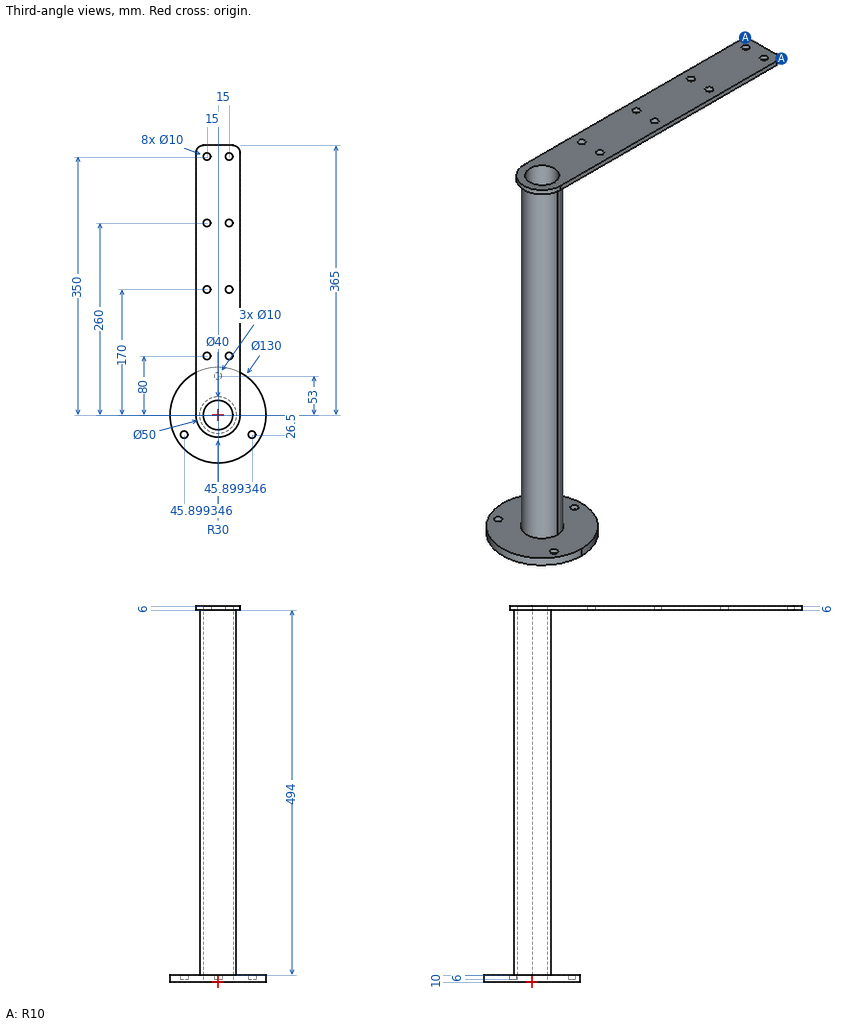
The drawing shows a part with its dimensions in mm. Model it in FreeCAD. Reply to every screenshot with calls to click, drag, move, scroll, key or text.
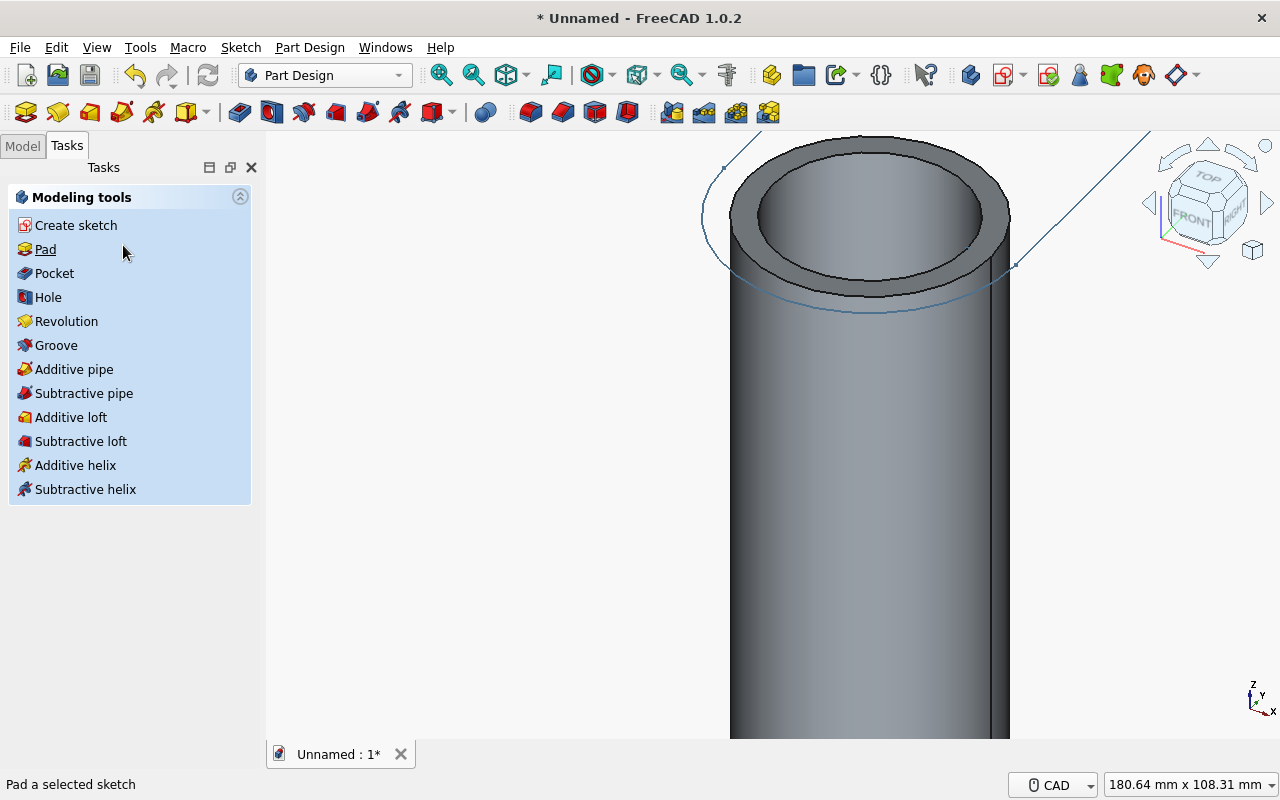
click(26, 112)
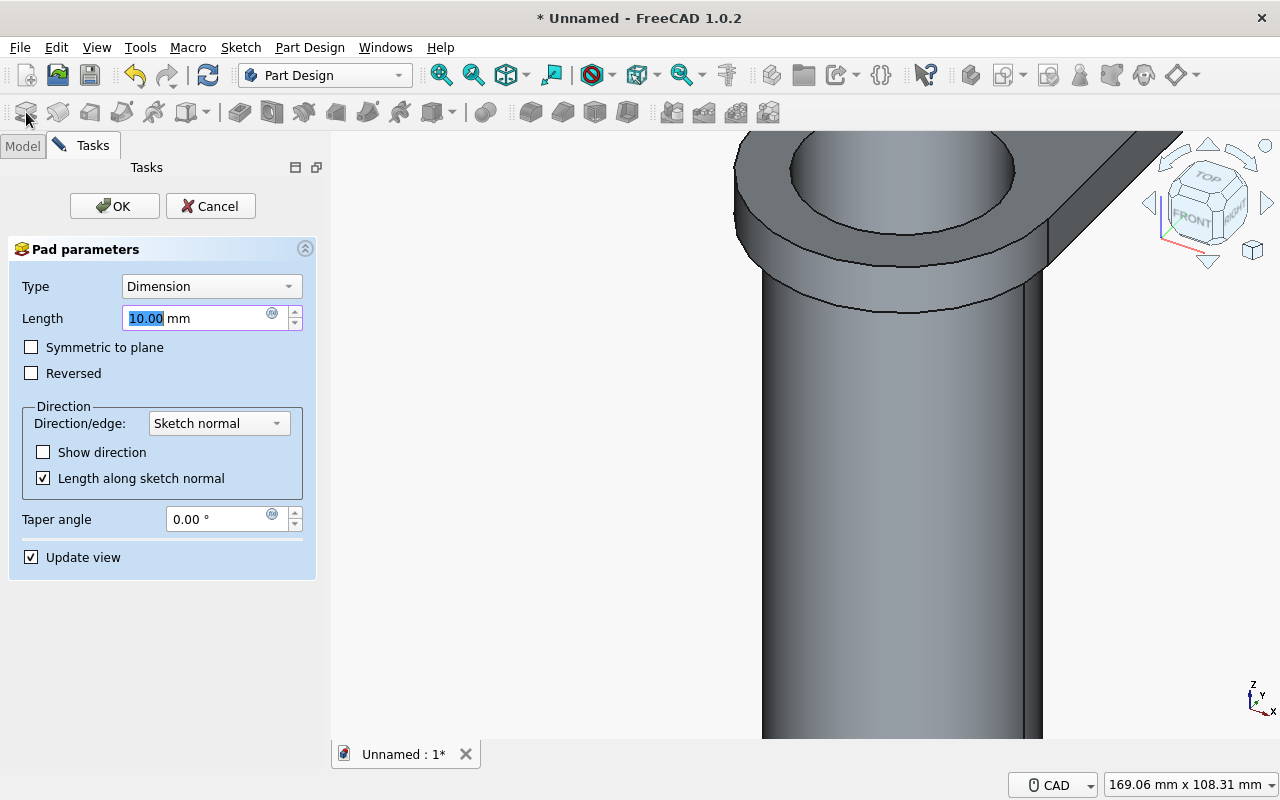
text(6)
key(Tab)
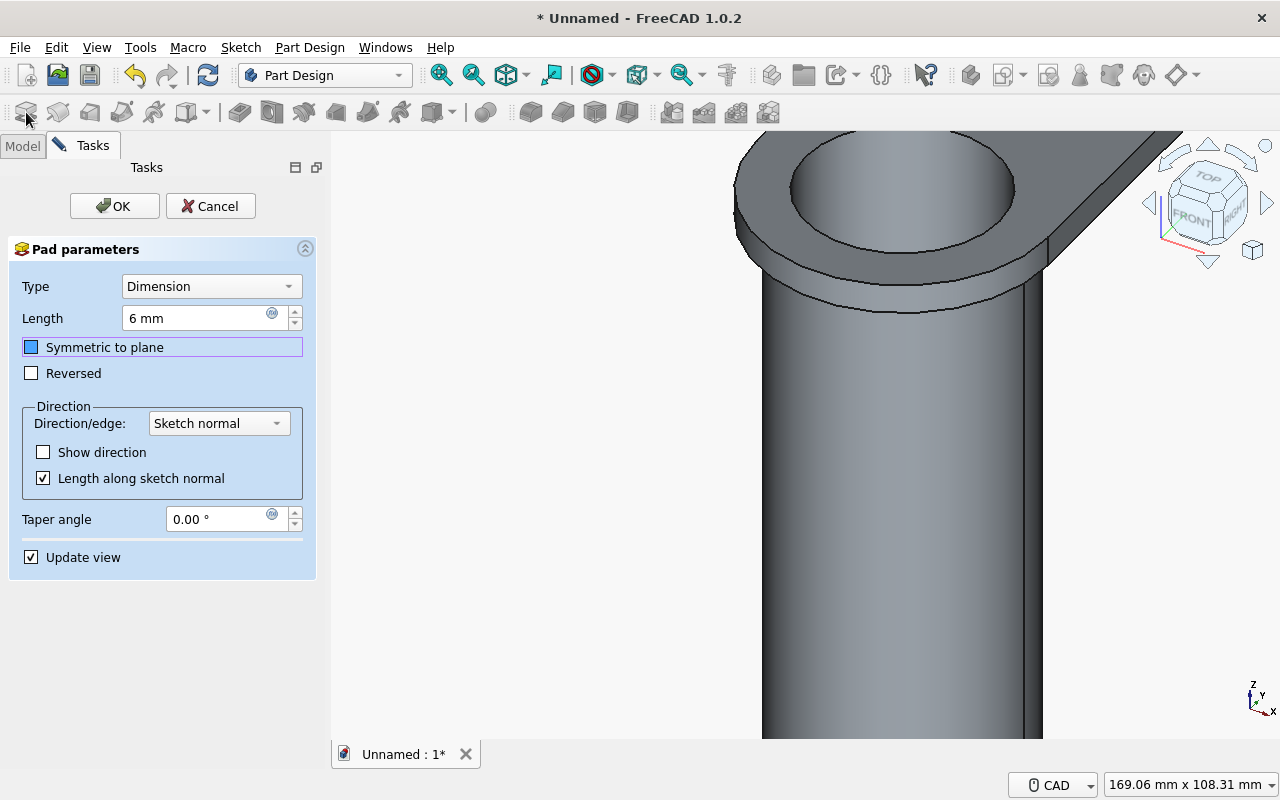
click(115, 206)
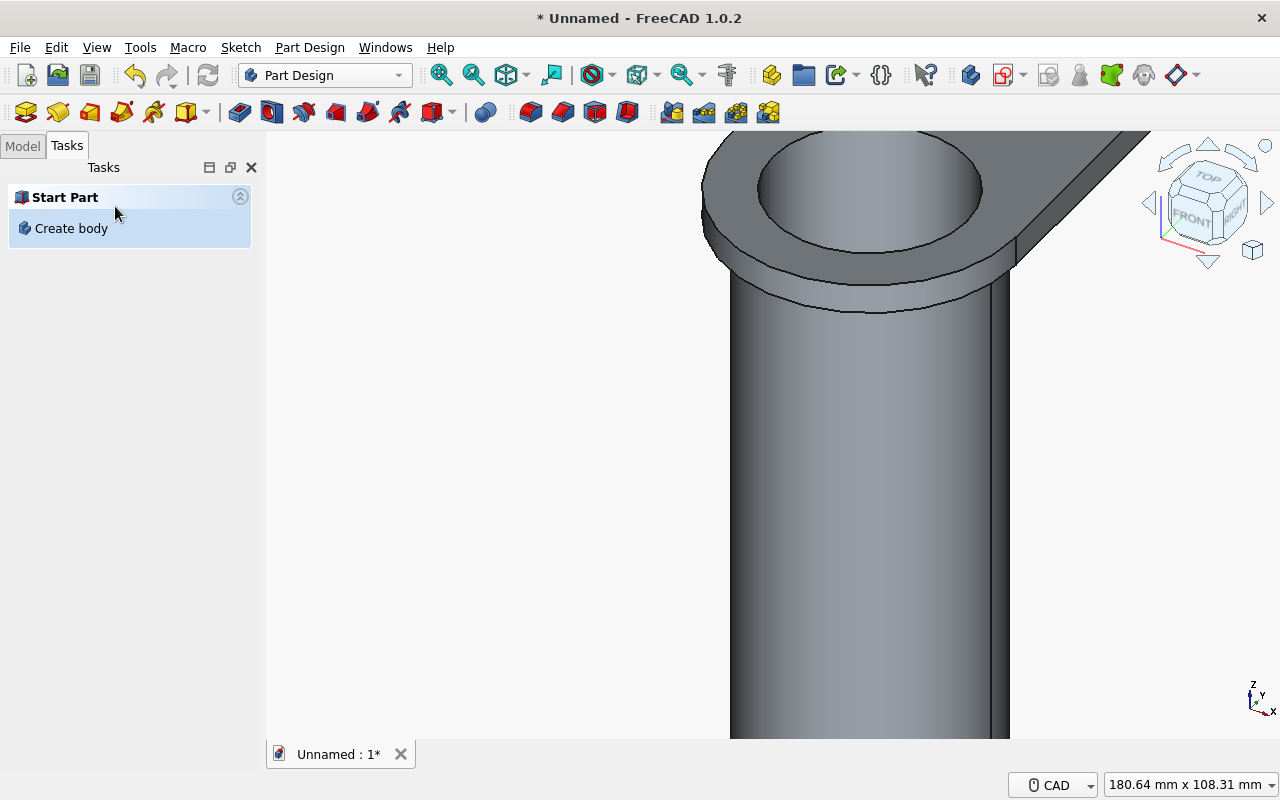
click(442, 76)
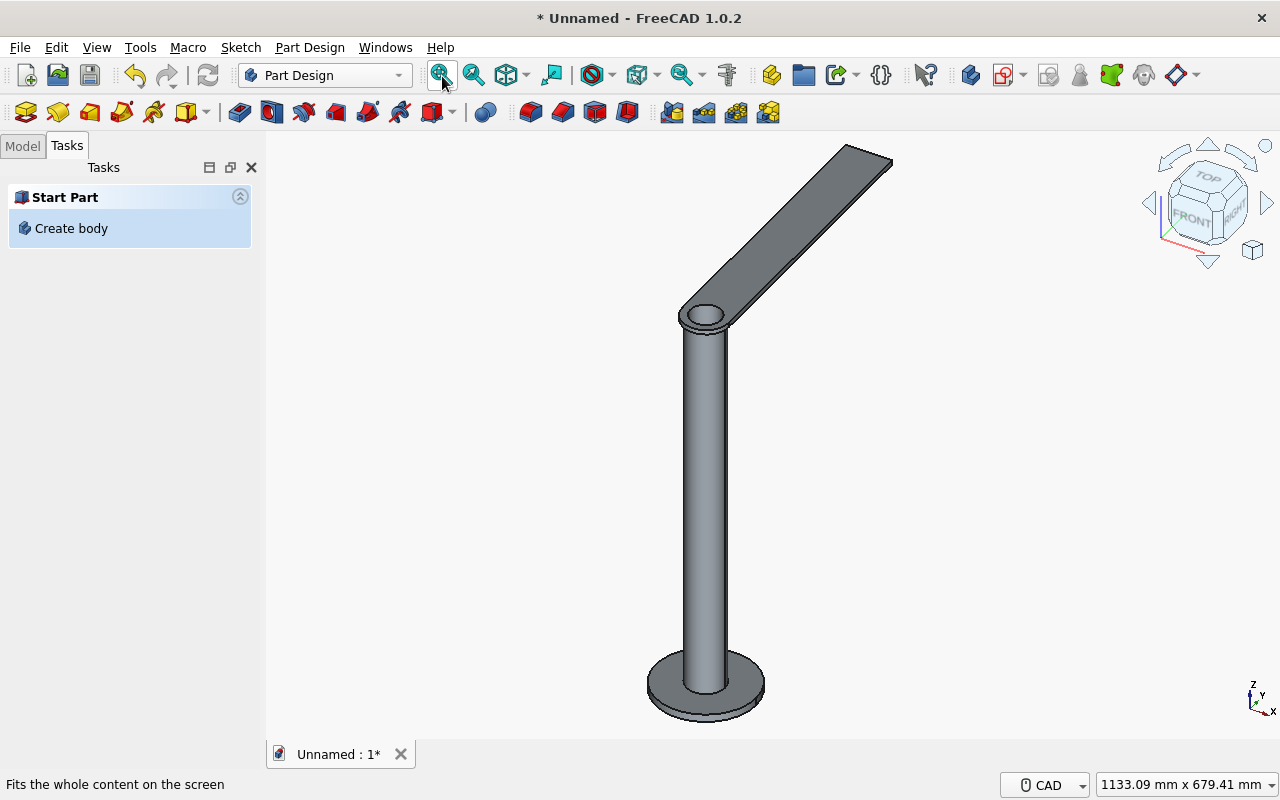
scroll(892, 161, up, 11)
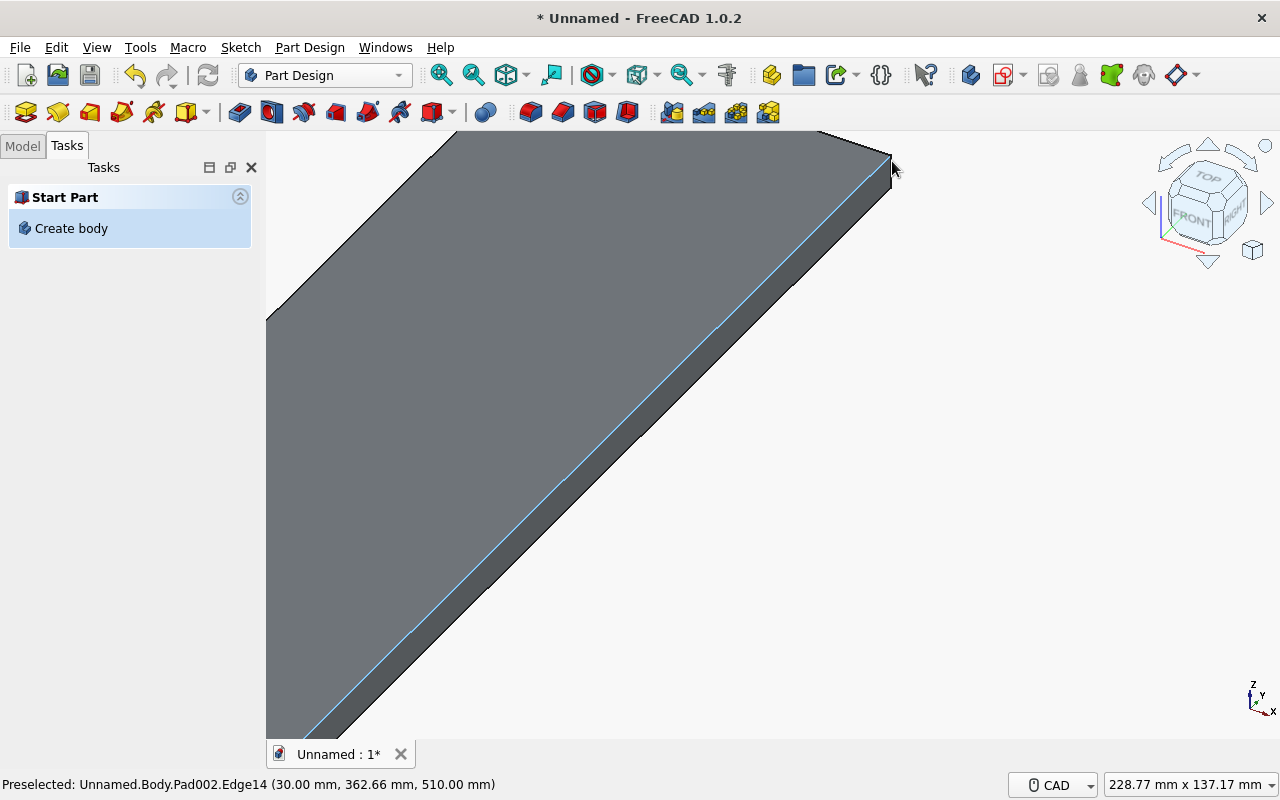
click(442, 76)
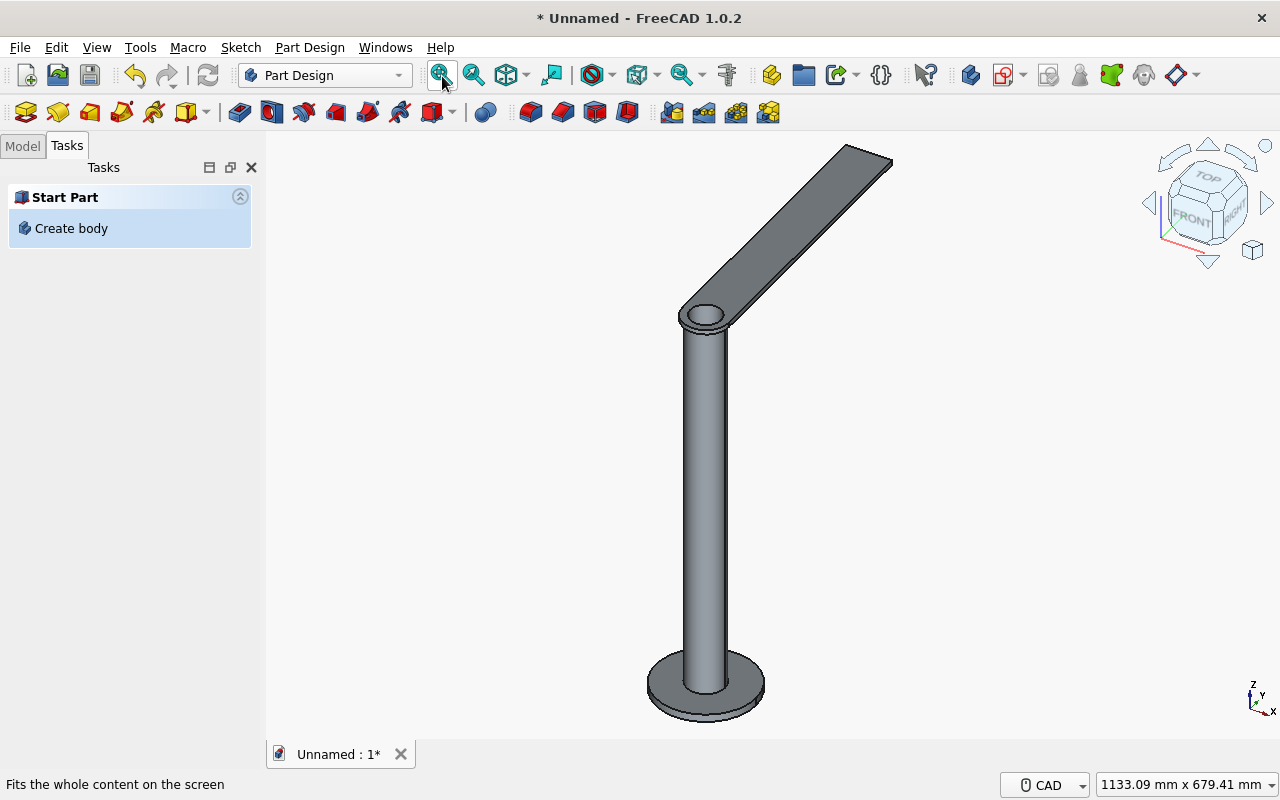
key(0)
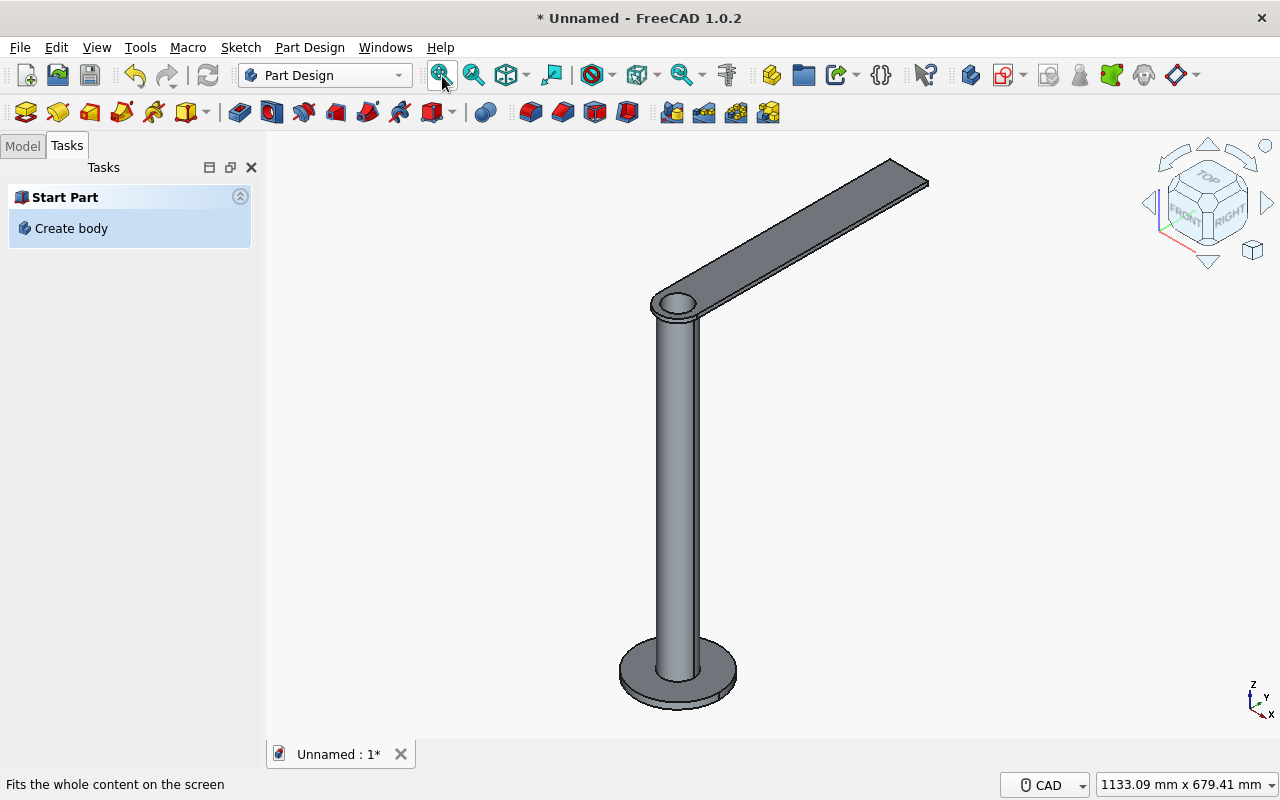
scroll(928, 182, up, 11)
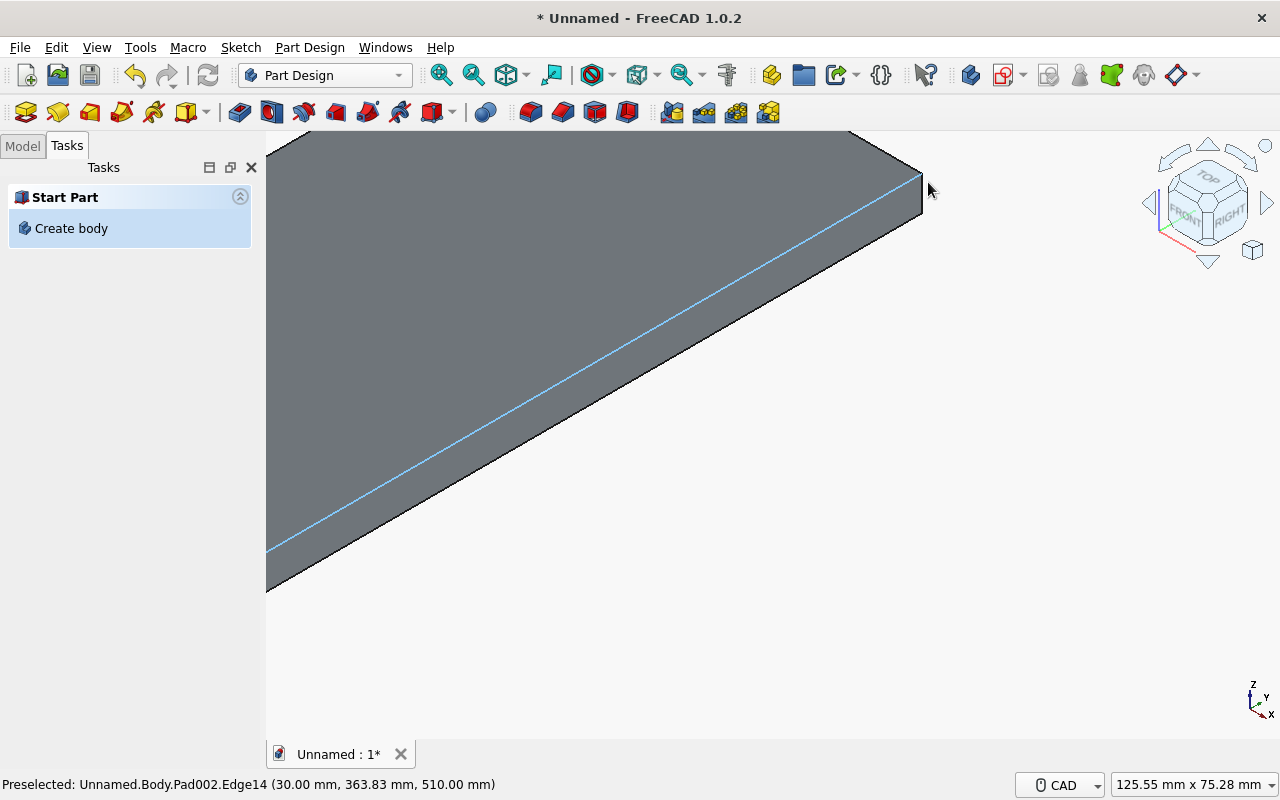
click(442, 76)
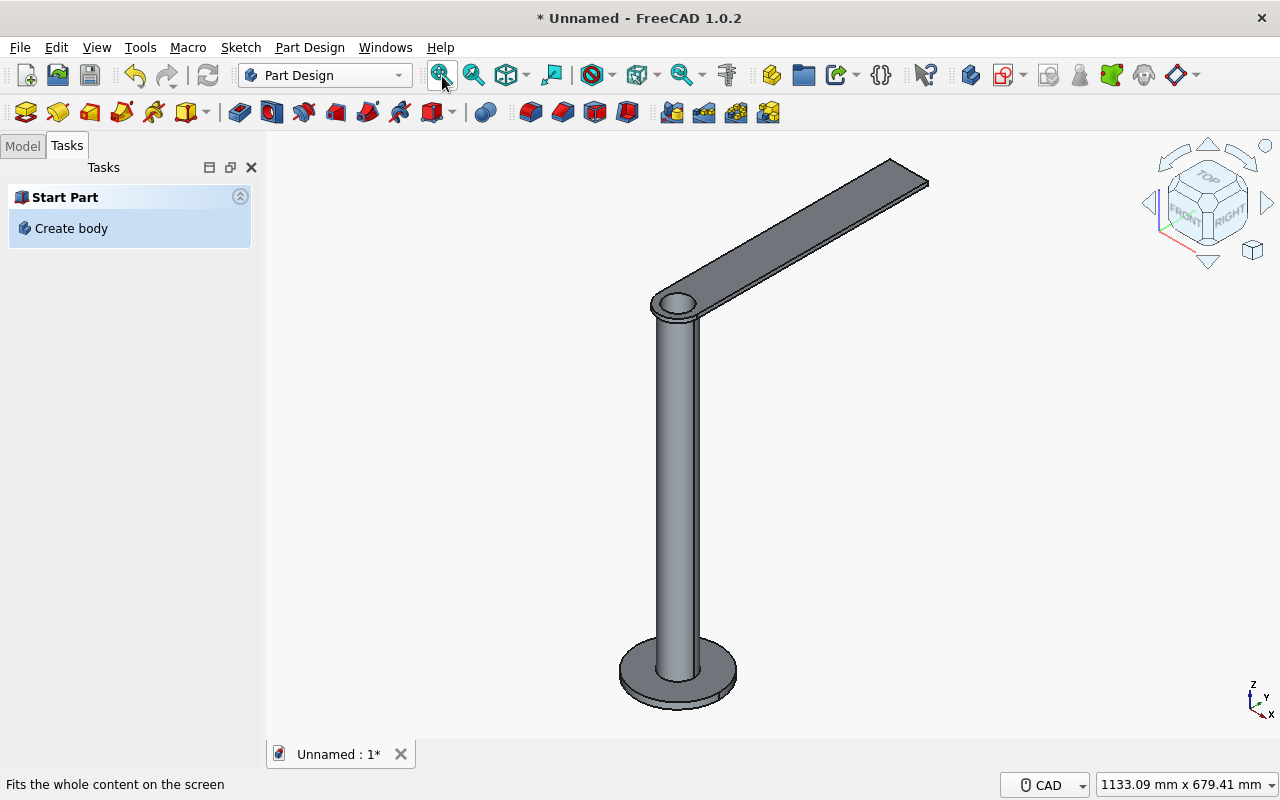
key(2)